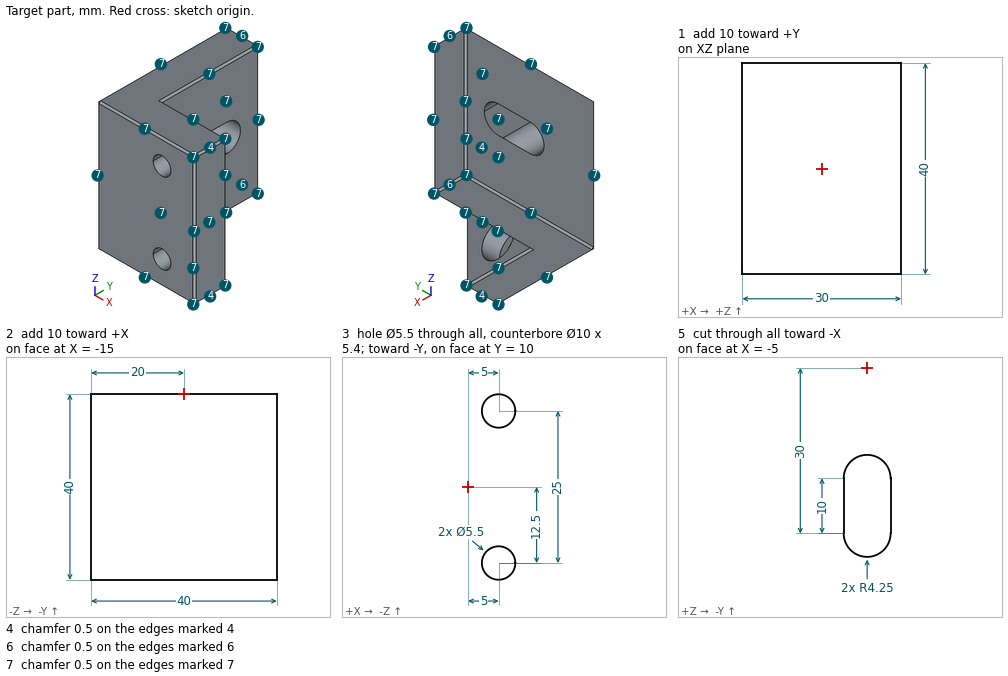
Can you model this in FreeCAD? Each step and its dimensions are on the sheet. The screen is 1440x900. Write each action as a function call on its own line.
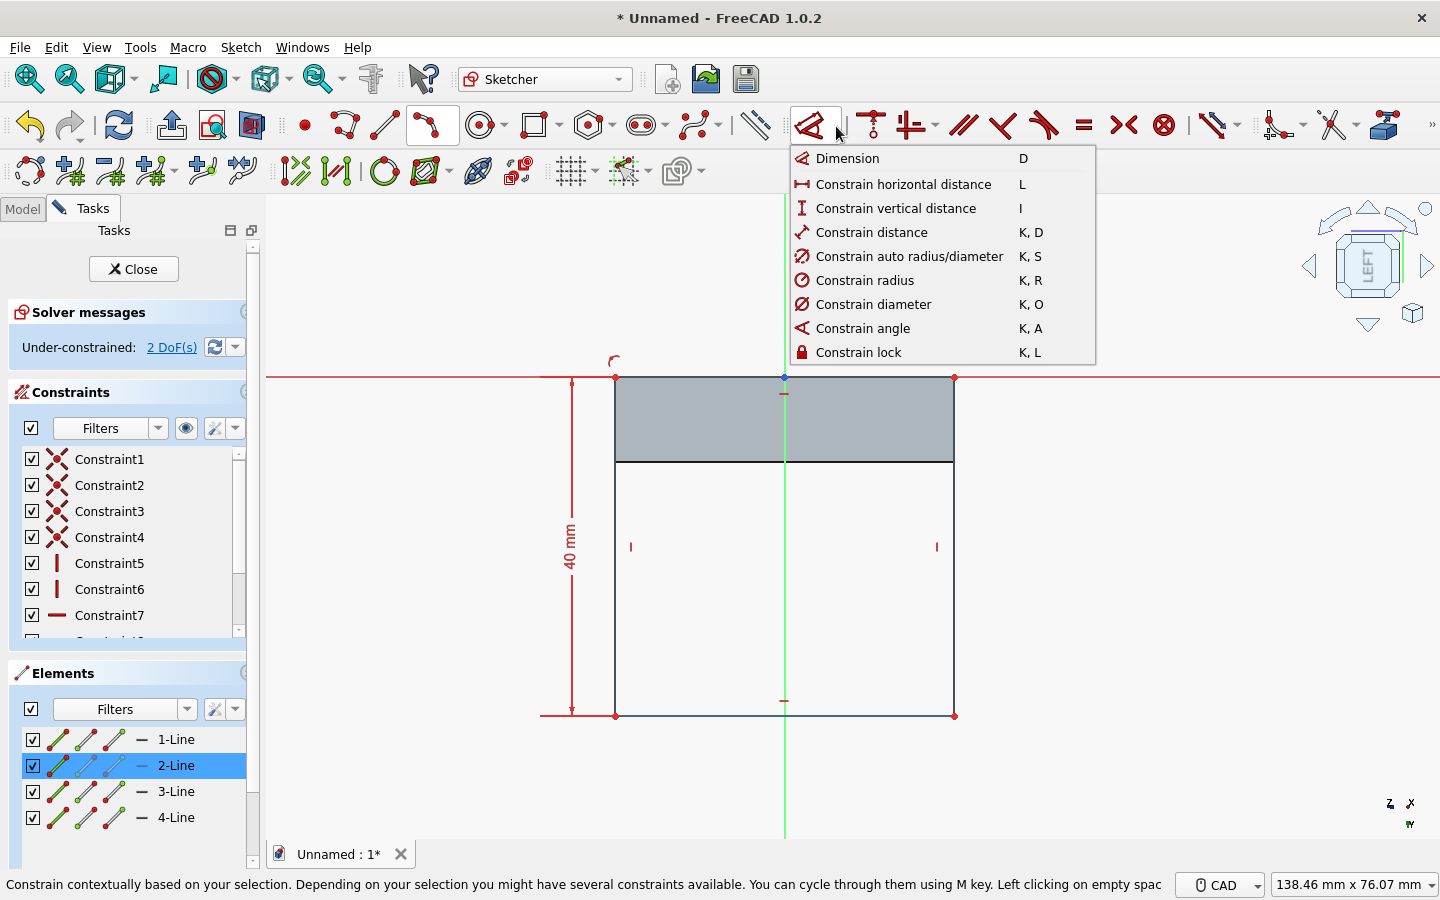
click(943, 184)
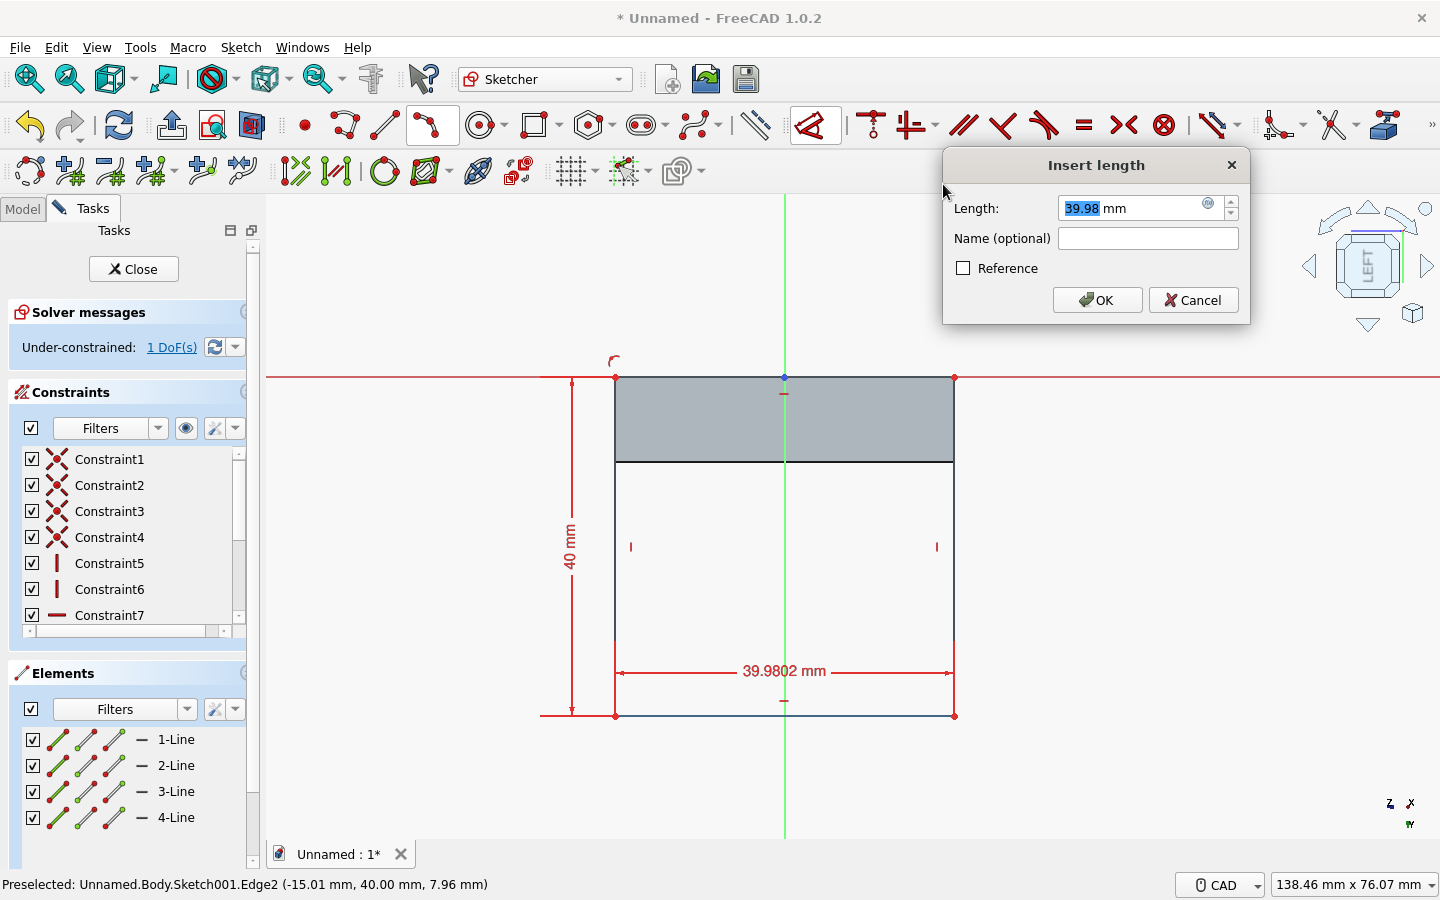
text(40)
key(Return)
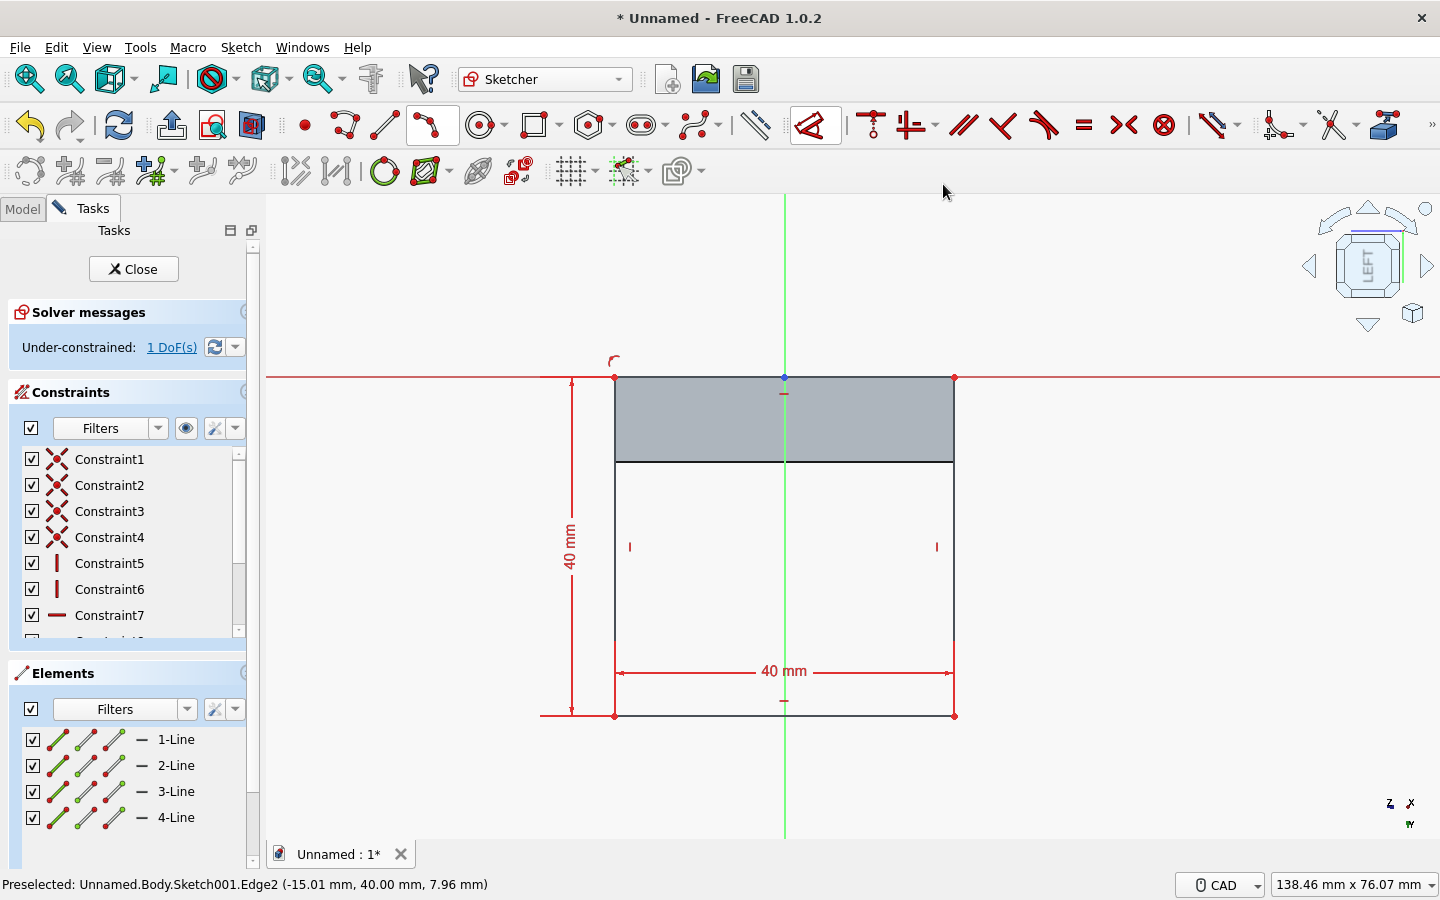
click(615, 377)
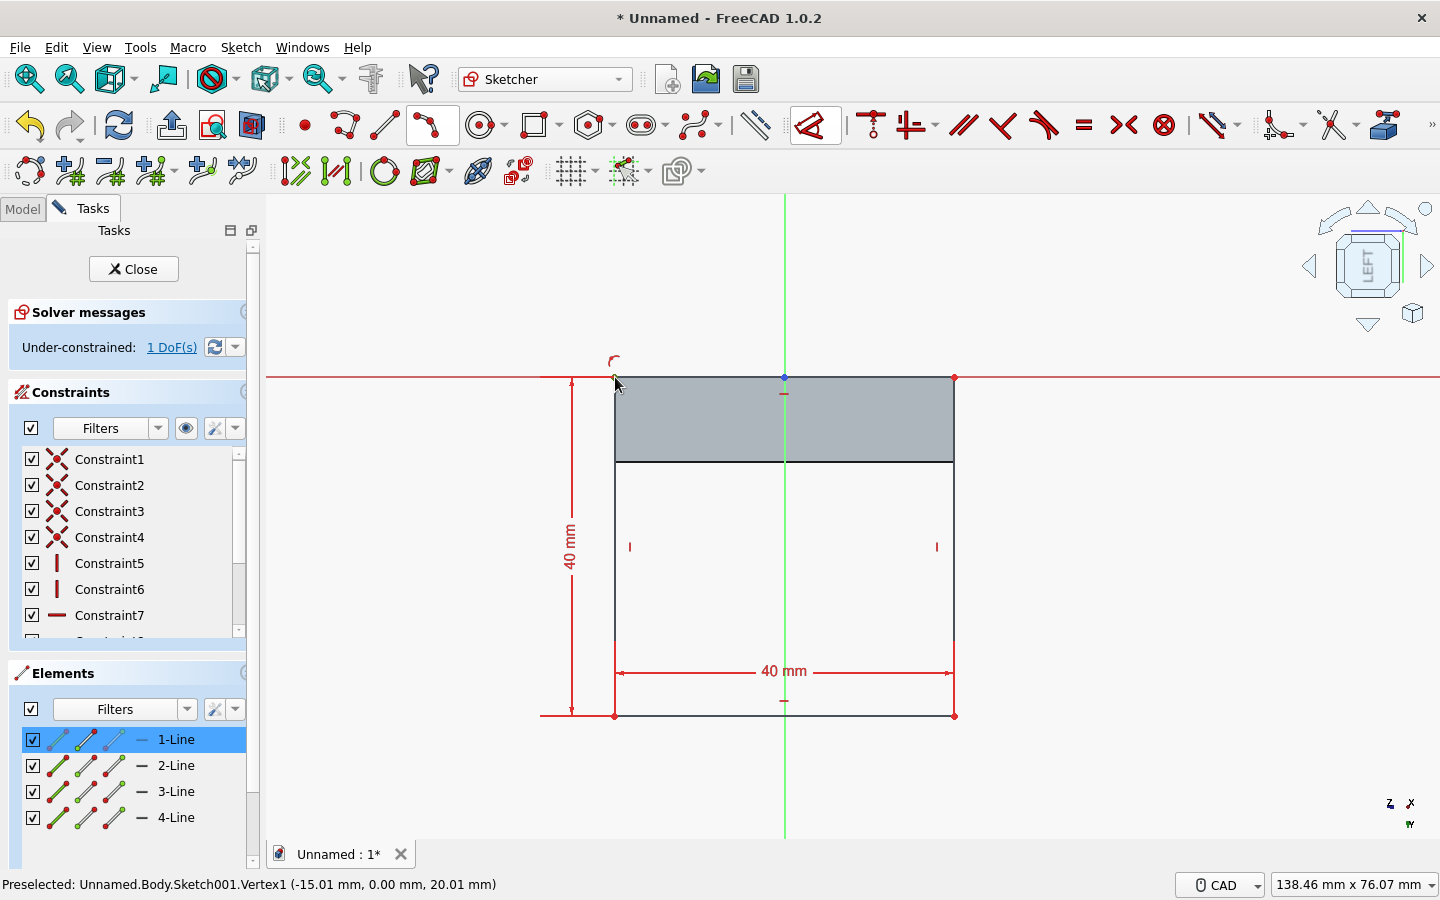
key(l)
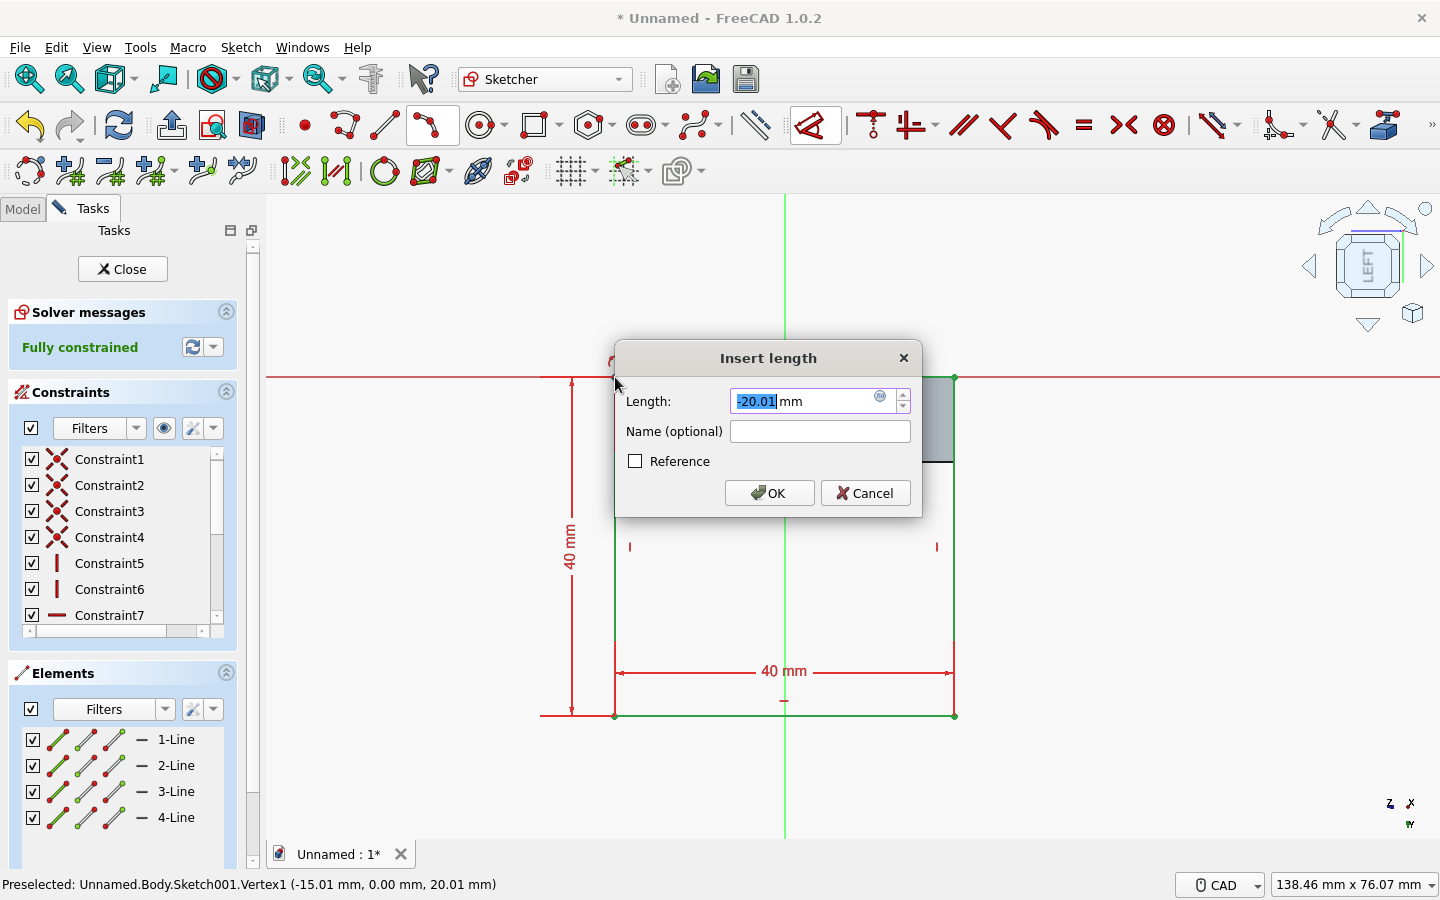
text(-20)
key(Return)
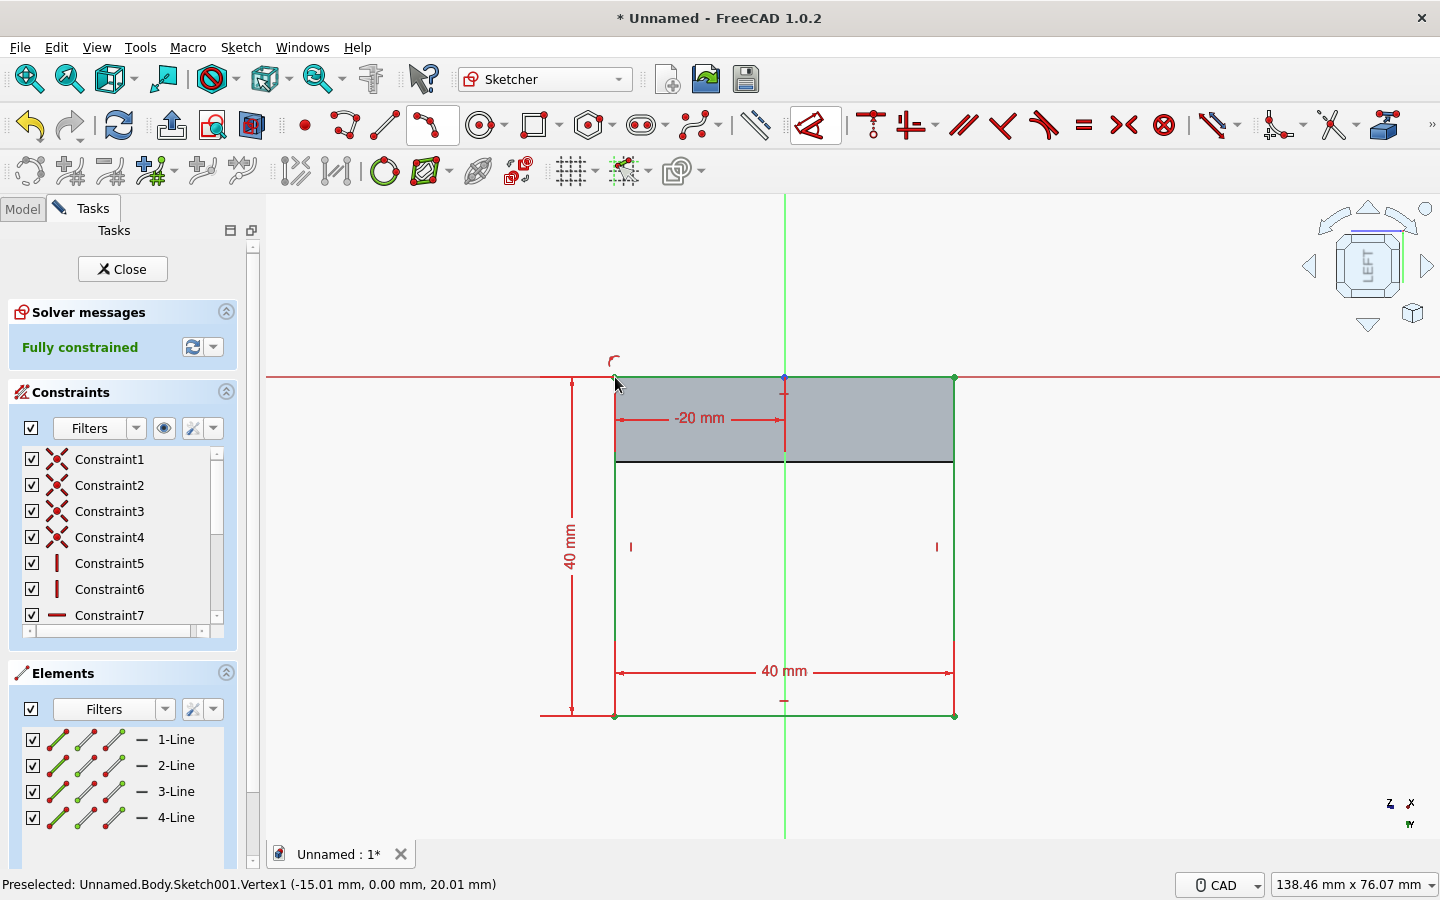
click(123, 269)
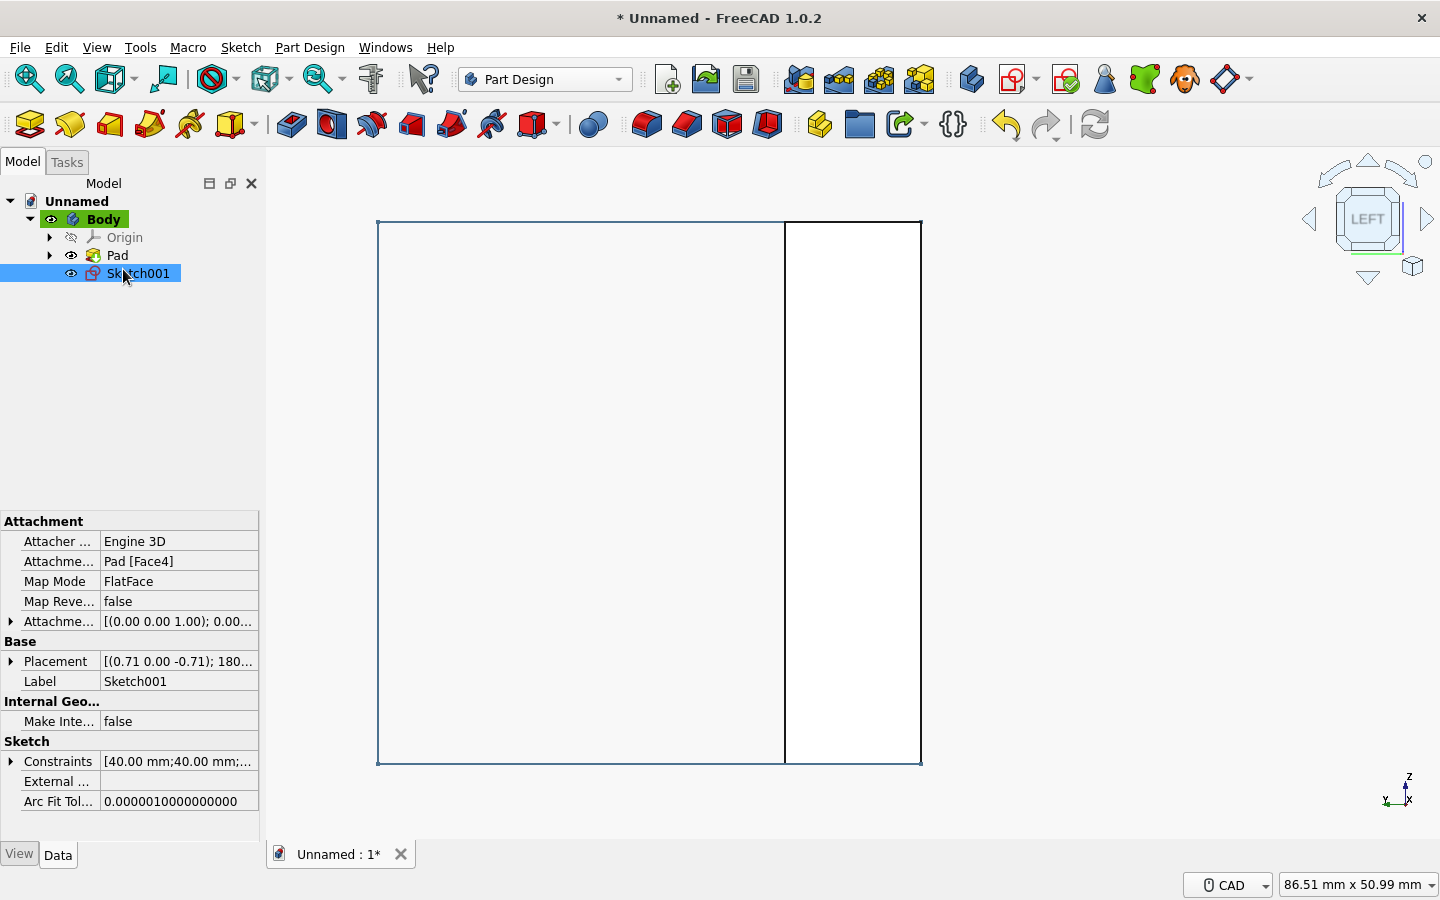
click(30, 124)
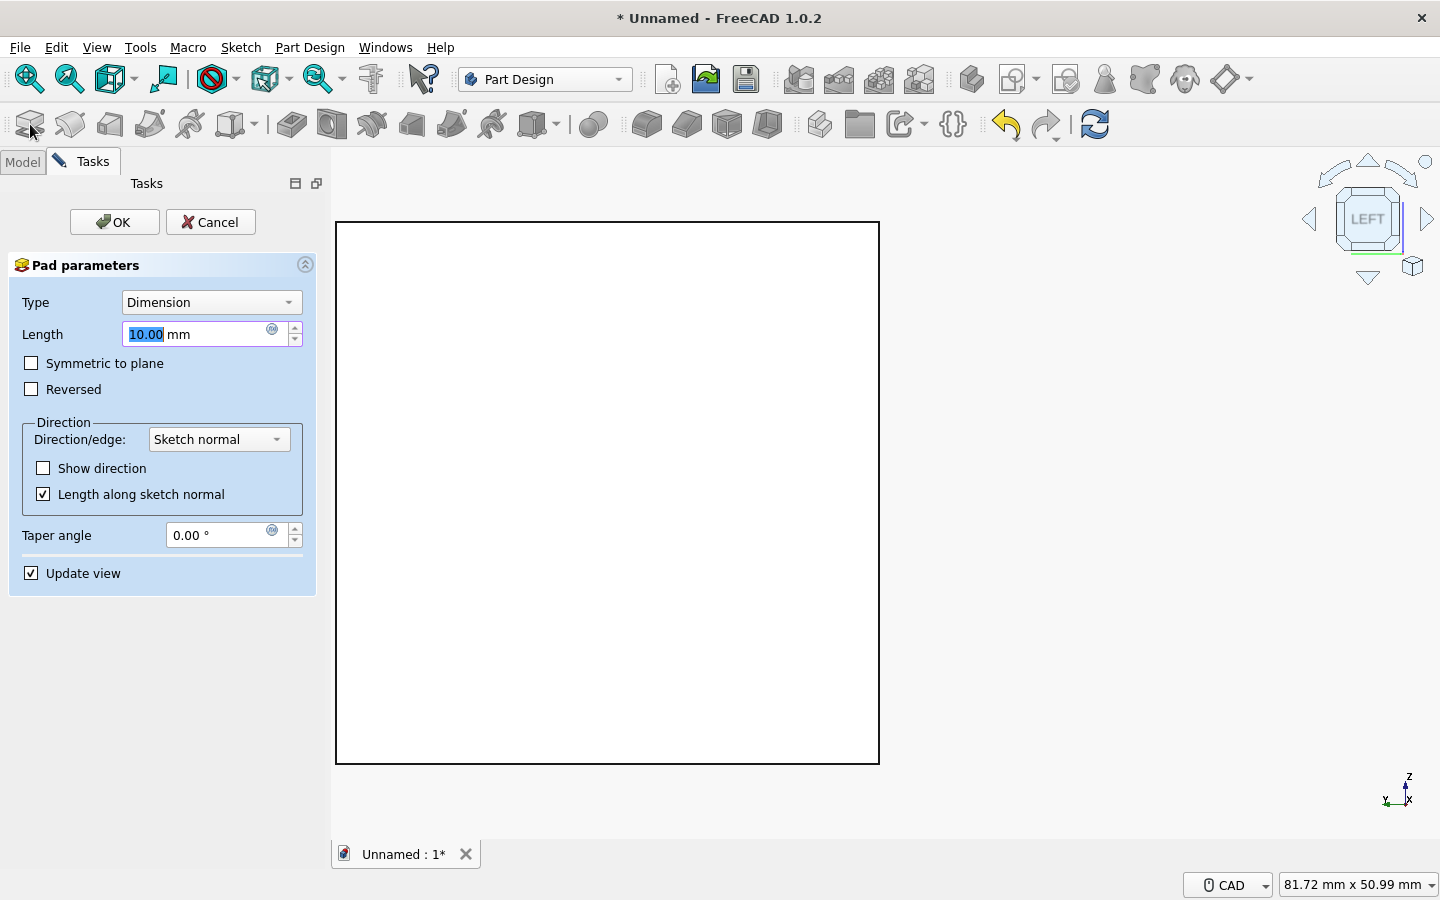
text(10)
key(Tab)